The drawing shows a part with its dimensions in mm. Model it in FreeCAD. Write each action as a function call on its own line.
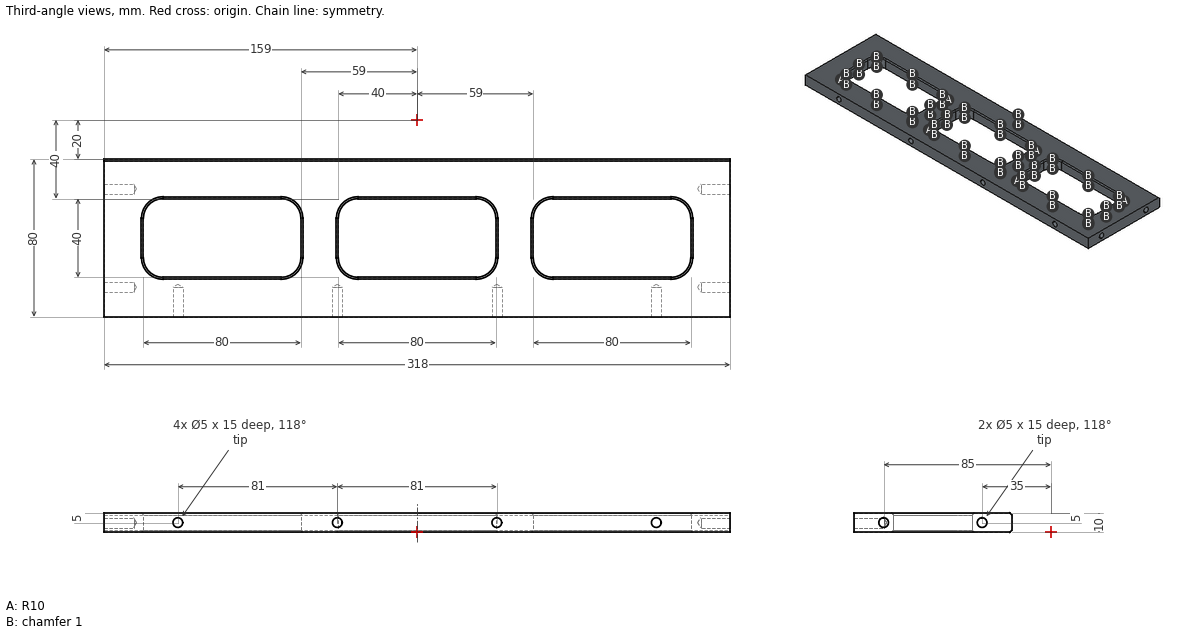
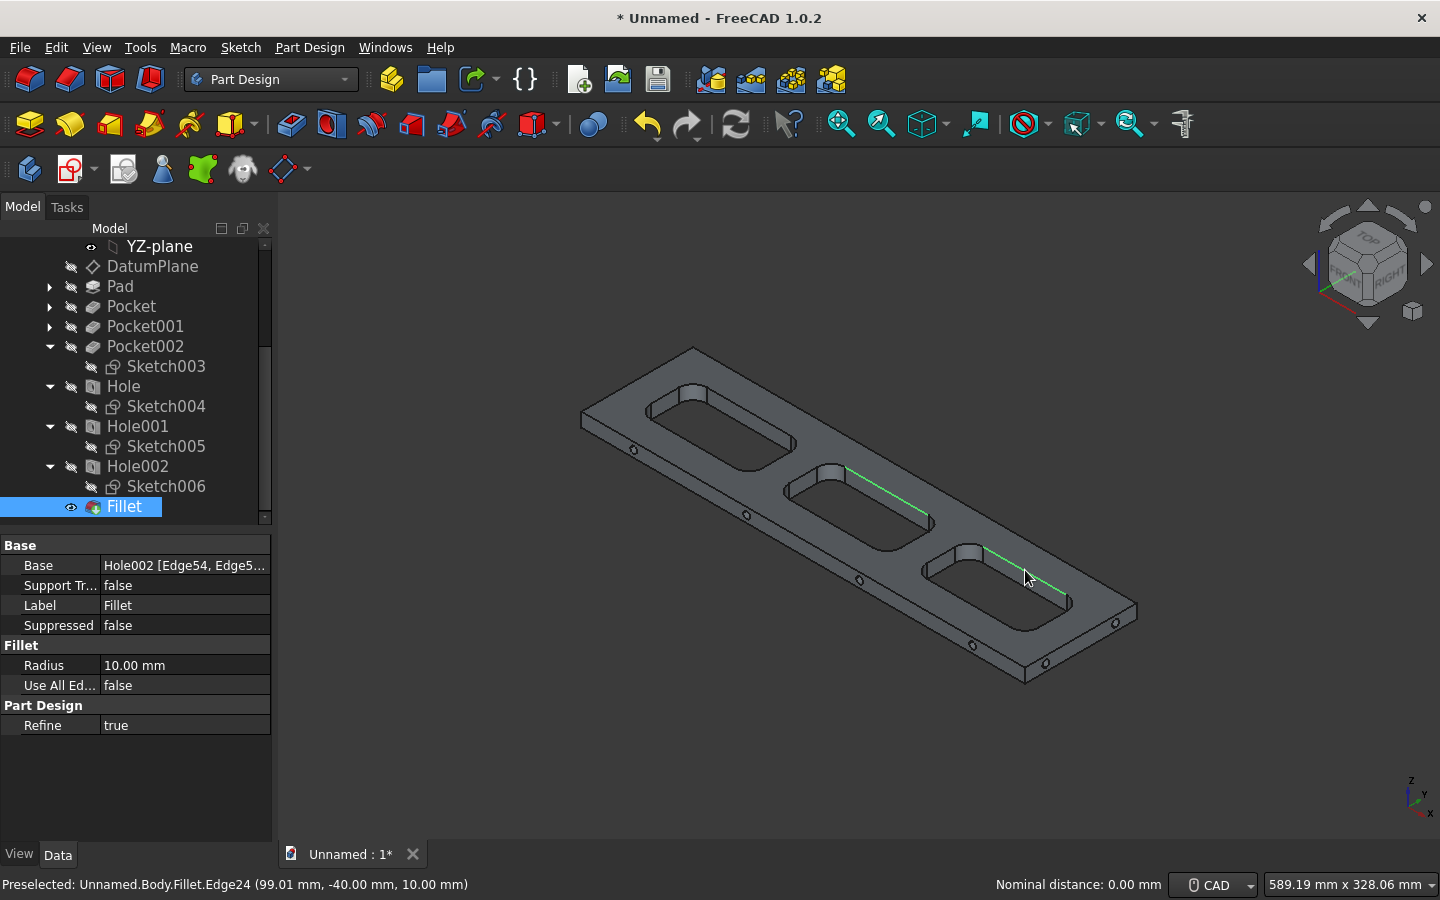
click(803, 474, ctrl)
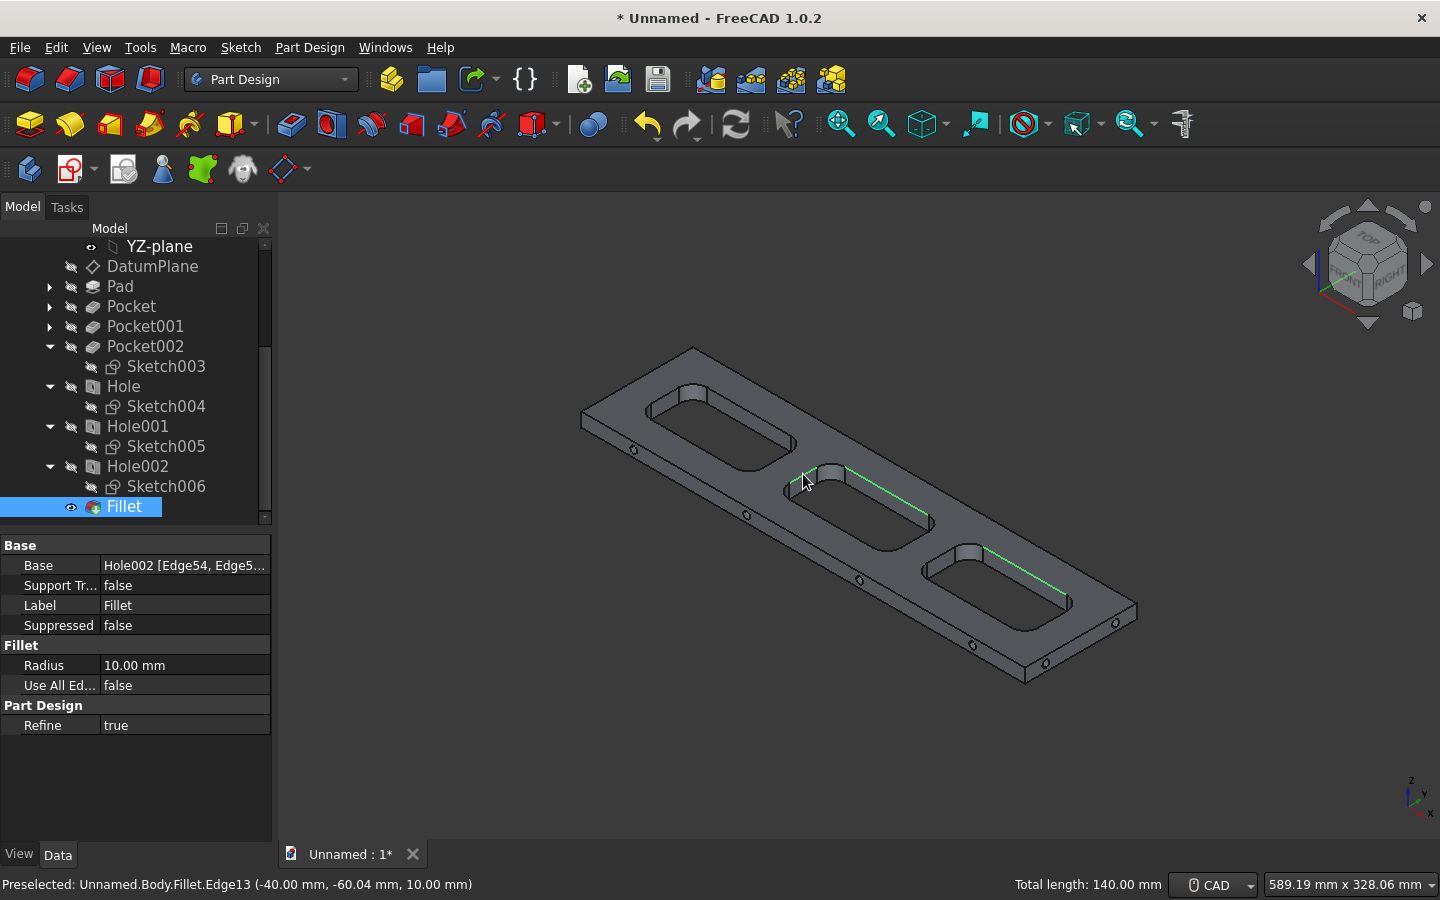
click(749, 411, ctrl)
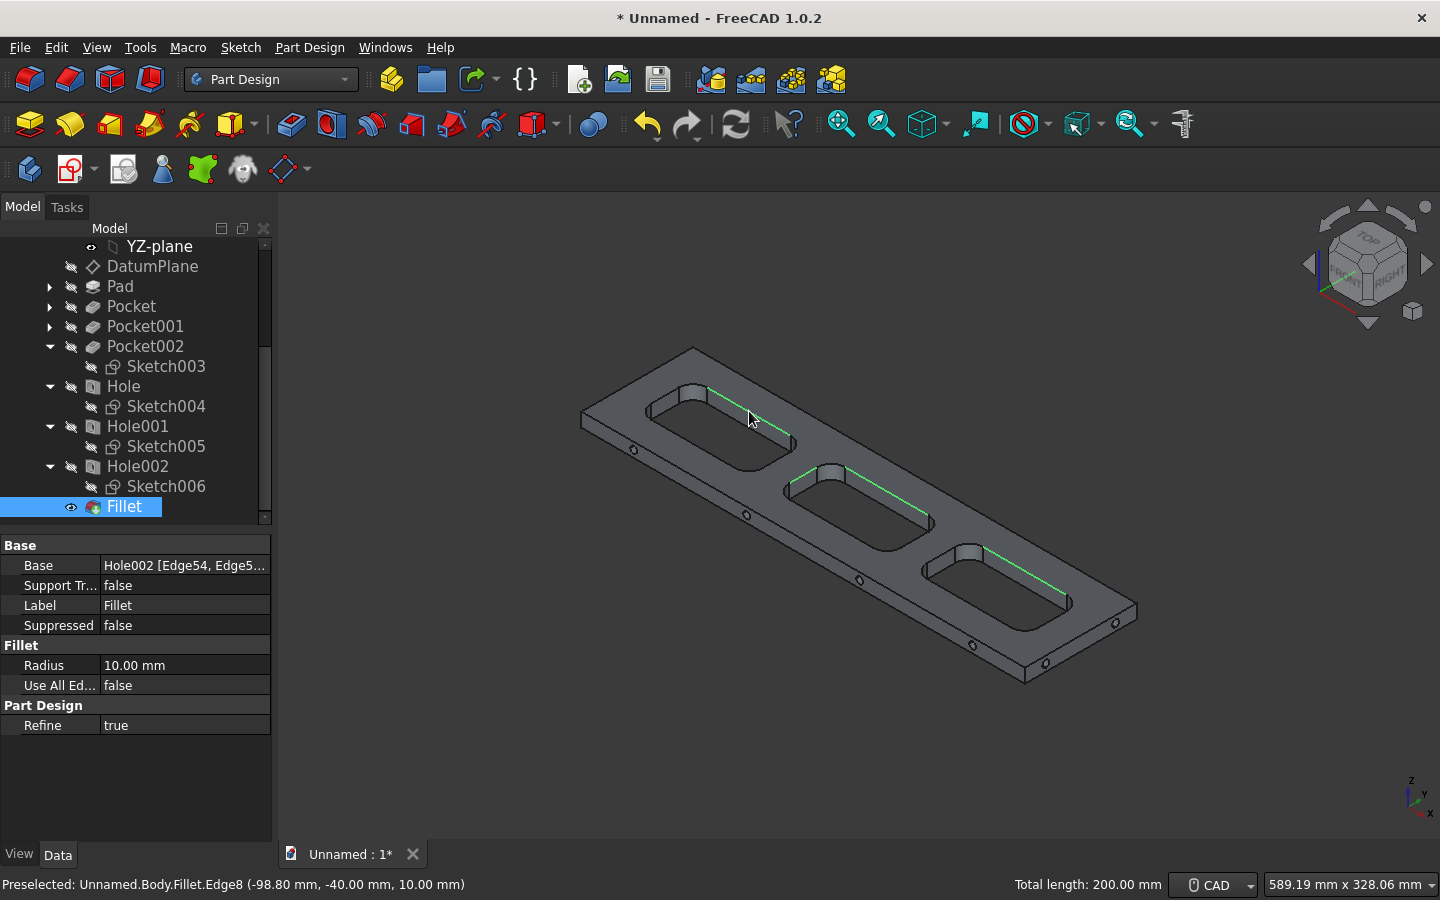
click(665, 395, ctrl)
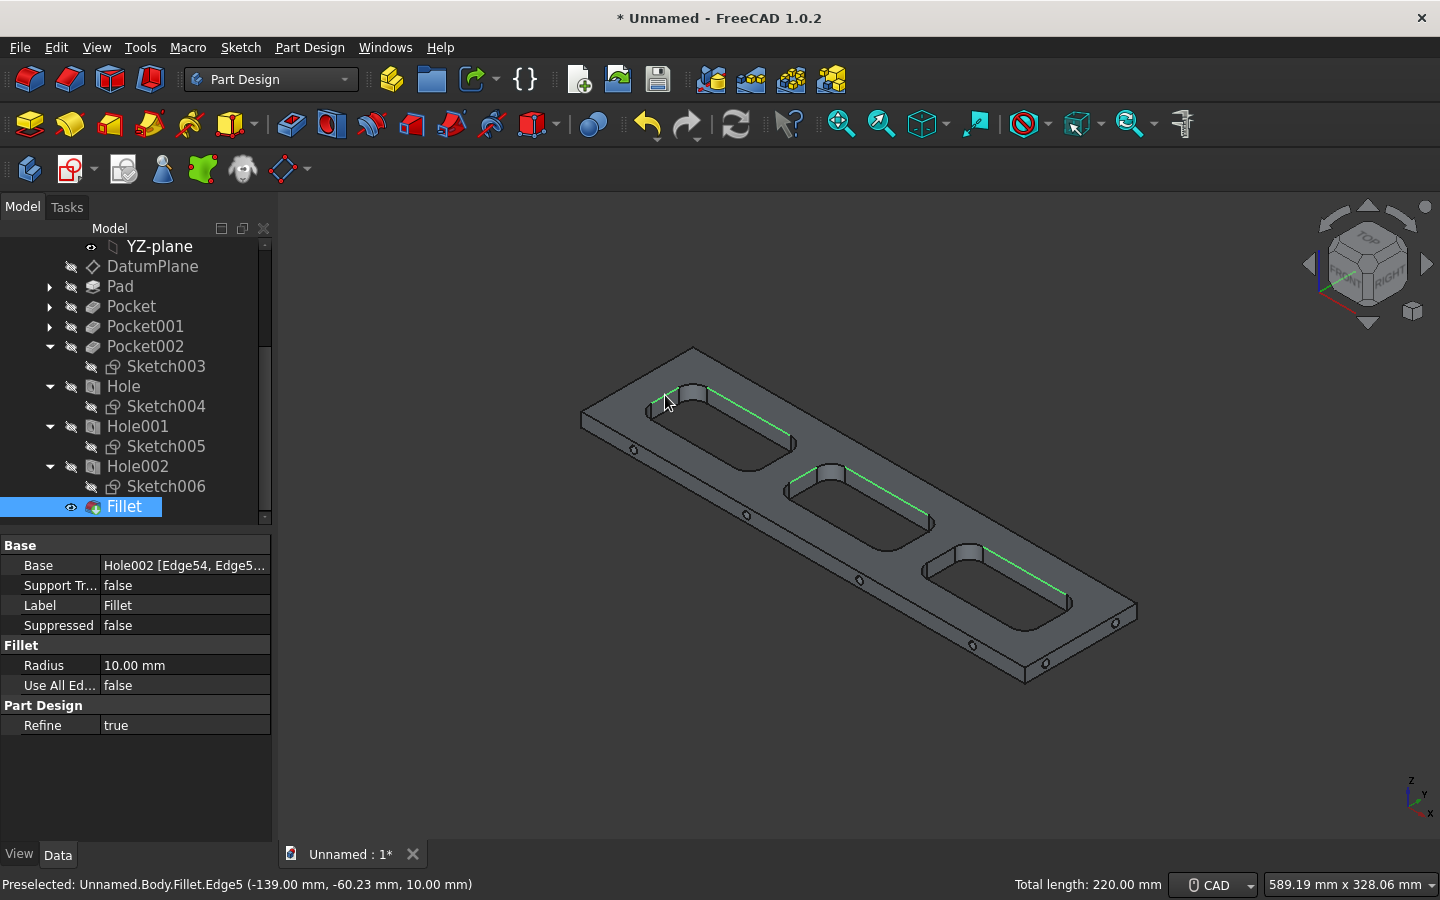
click(941, 554, ctrl)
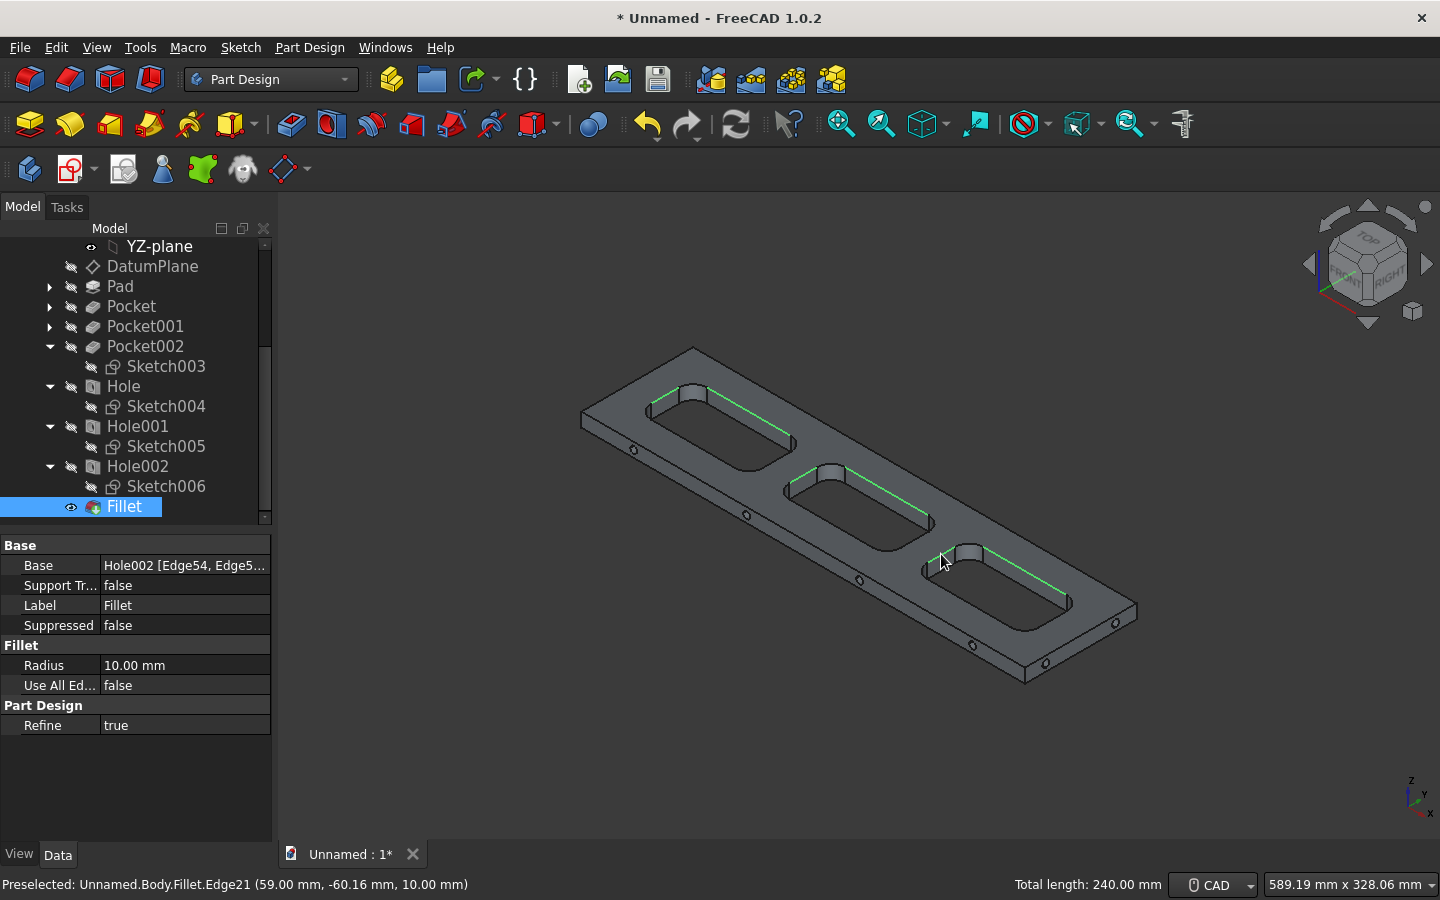
click(934, 521, ctrl)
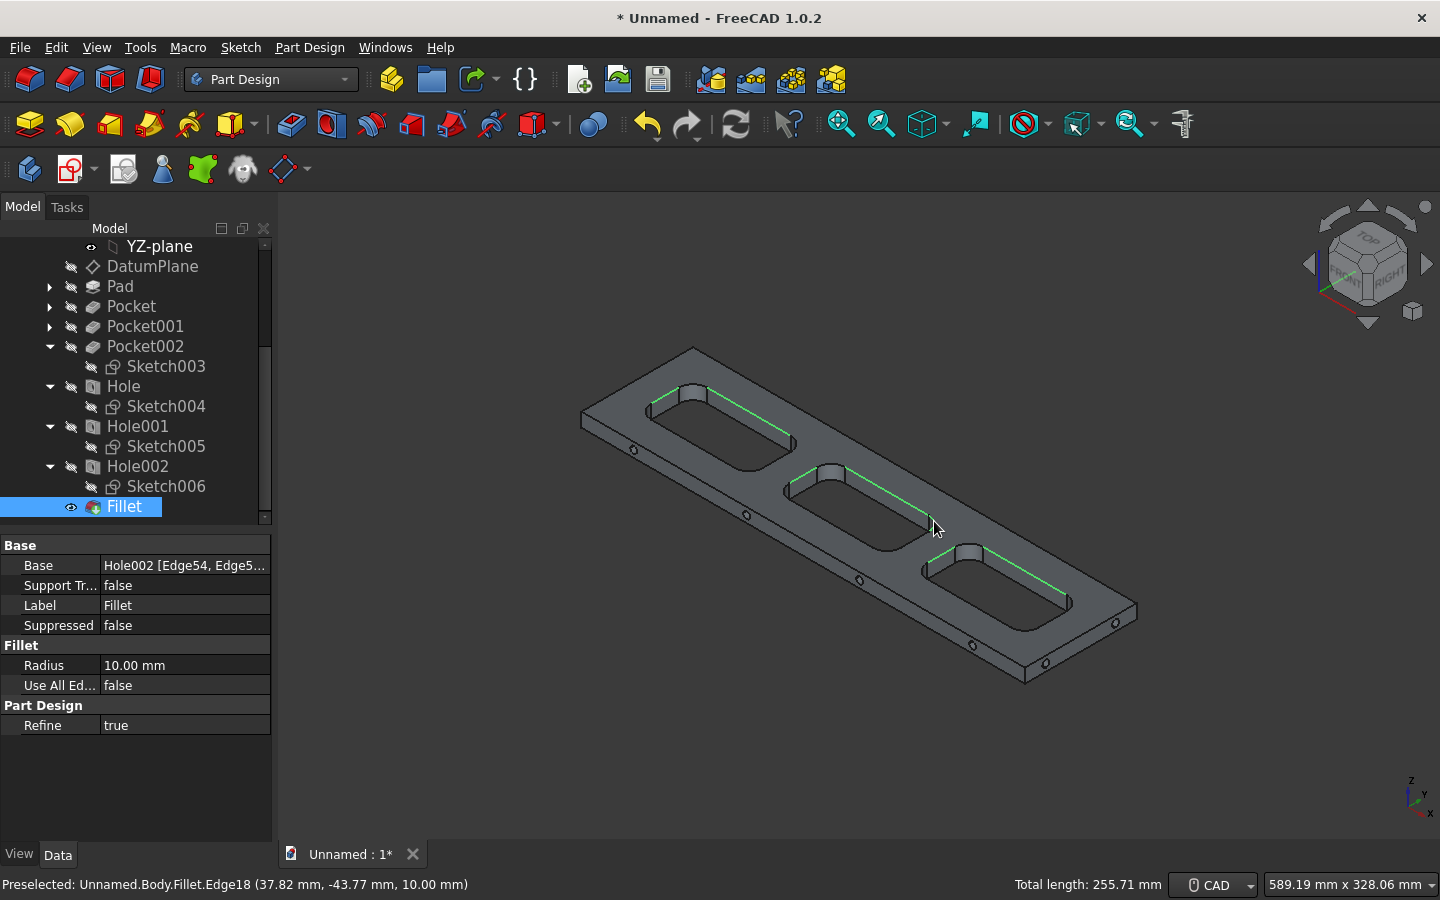
click(1073, 602, ctrl)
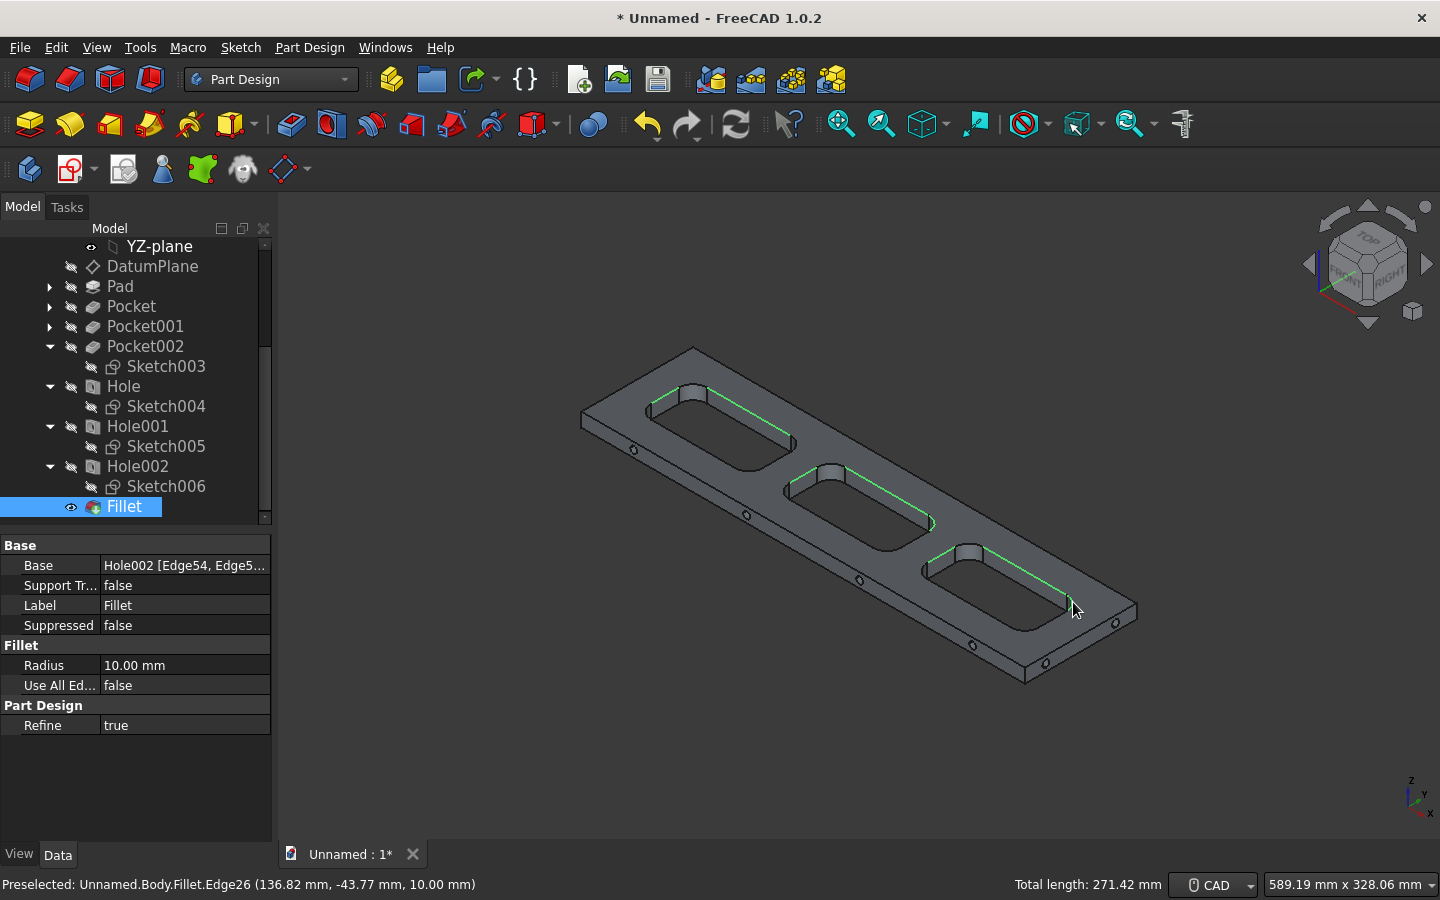
click(783, 490, ctrl)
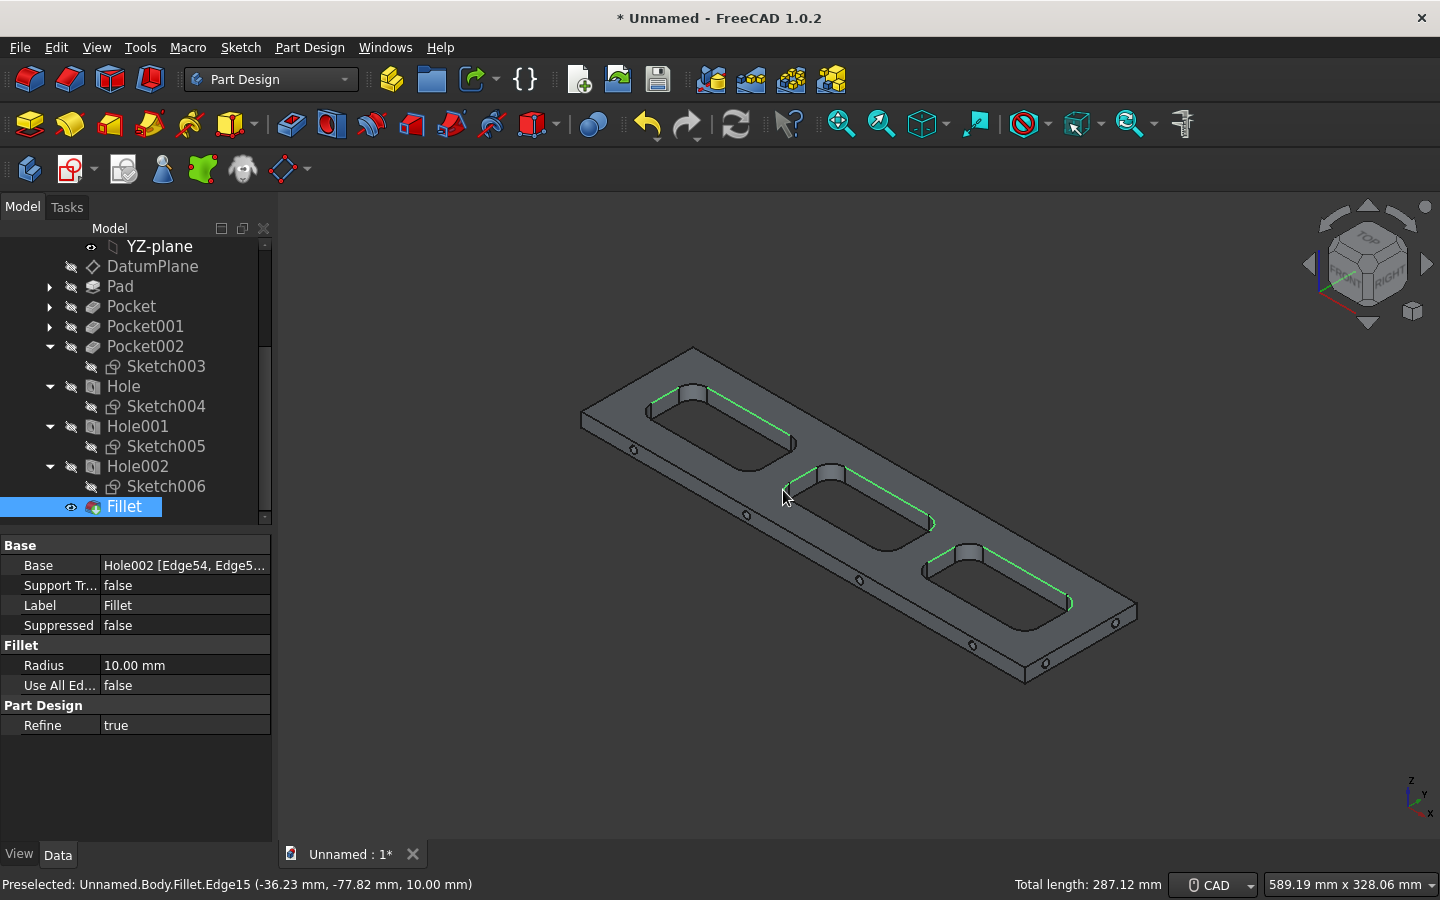
click(1012, 627, ctrl)